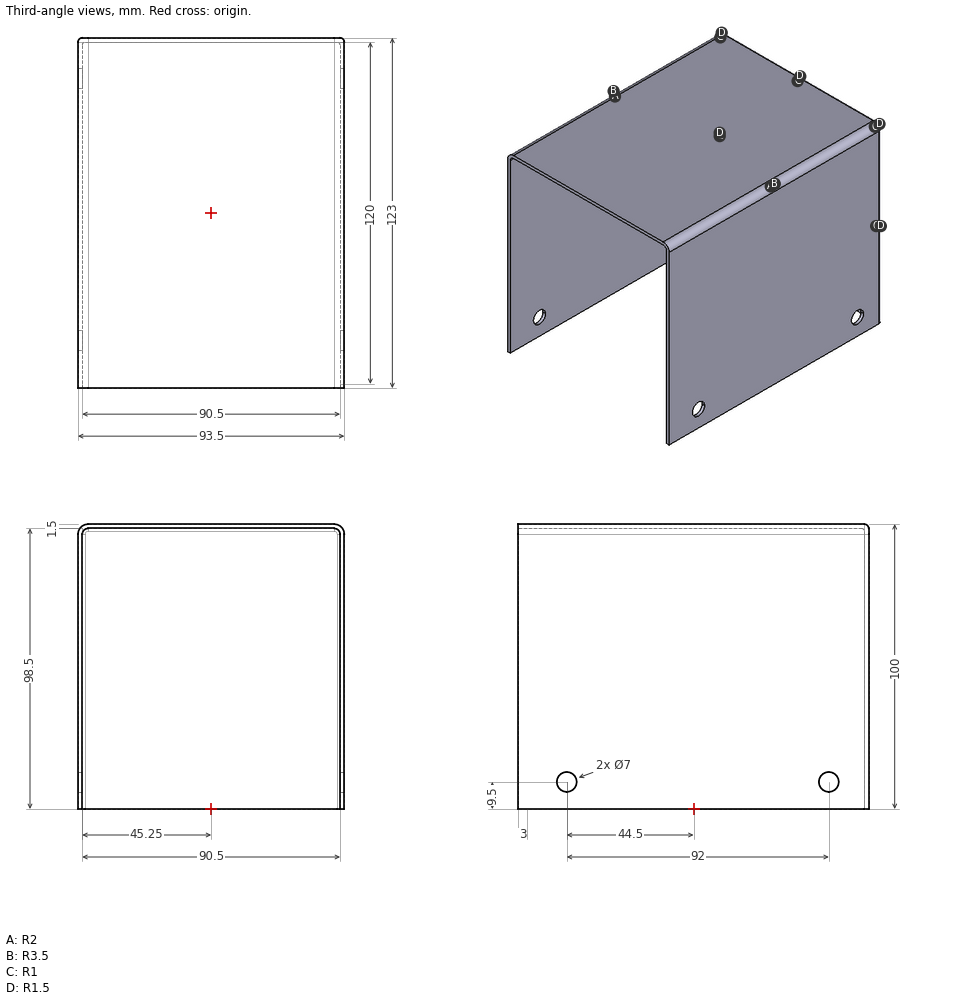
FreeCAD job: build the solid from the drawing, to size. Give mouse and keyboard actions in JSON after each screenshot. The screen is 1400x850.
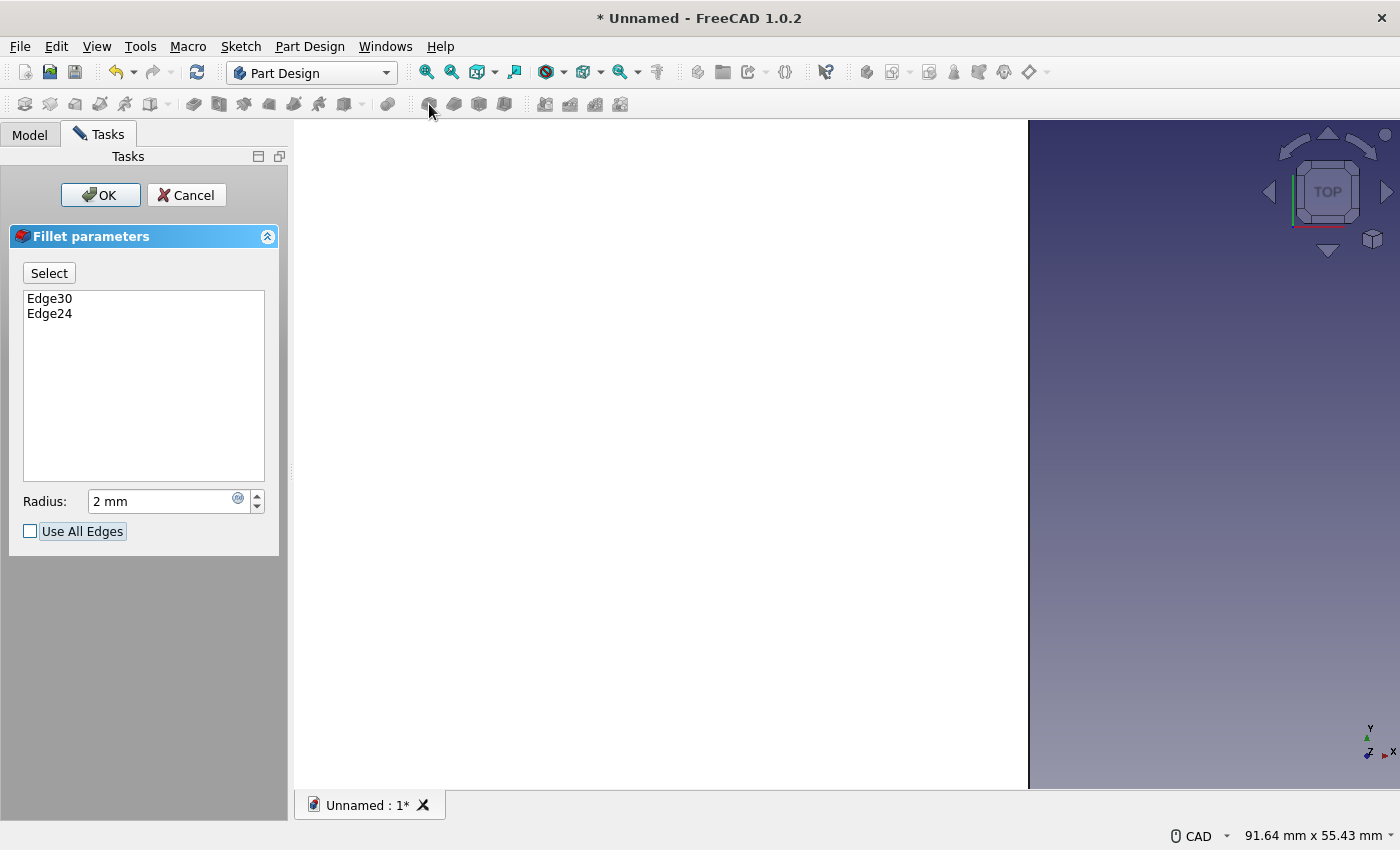
{"action": "left_click", "coordinate": [101, 195]}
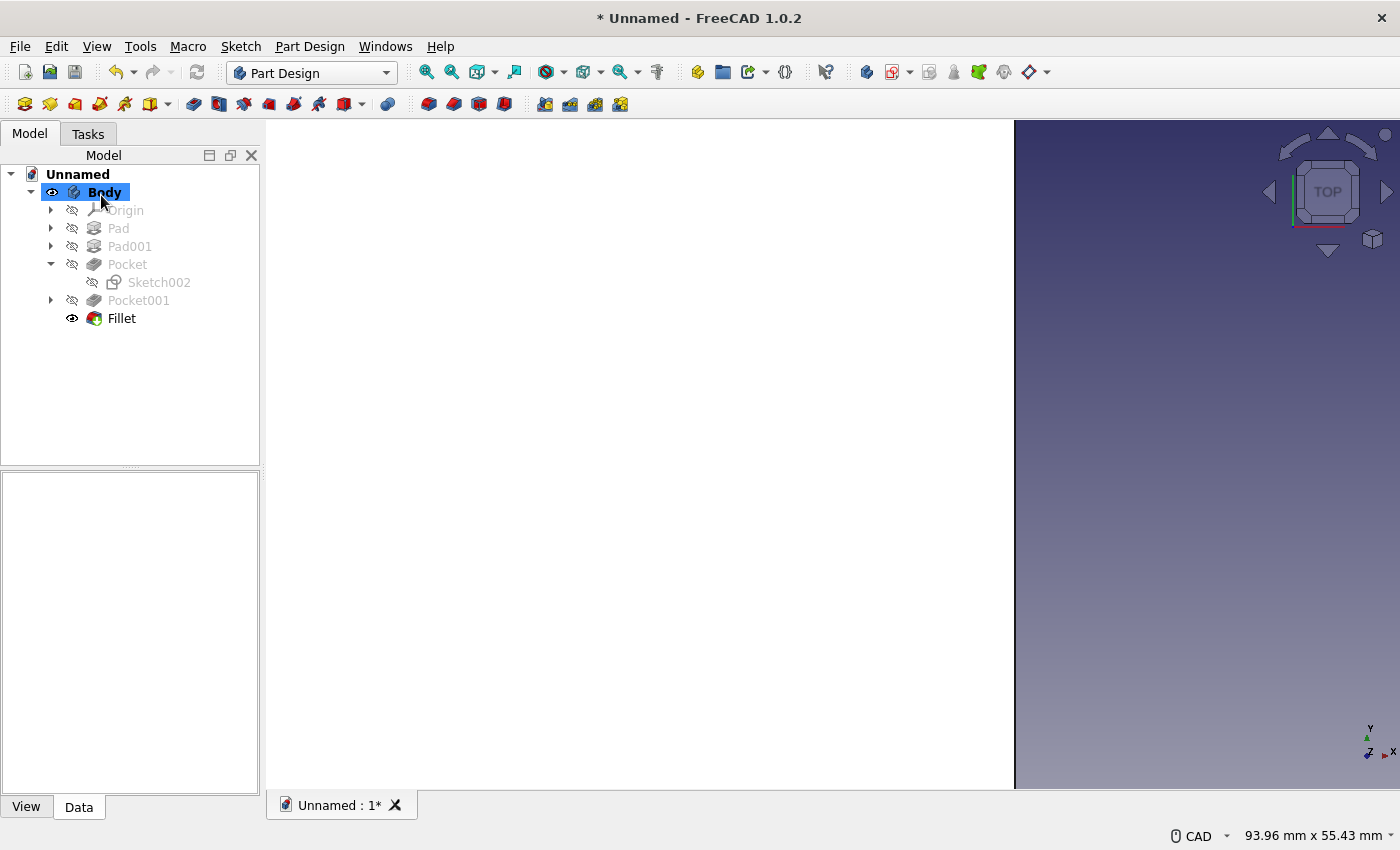
{"action": "left_click", "coordinate": [427, 72]}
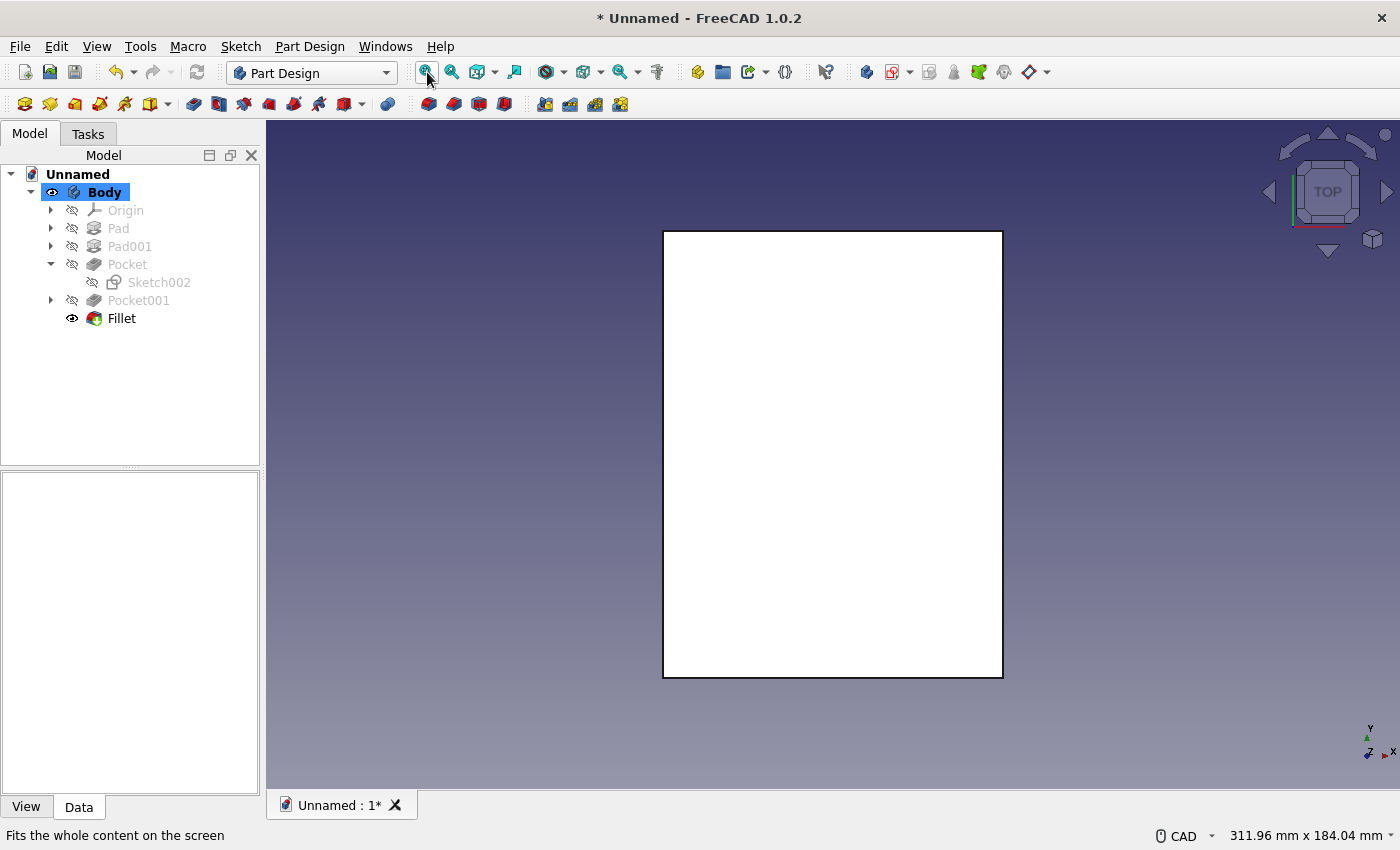
{"action": "left_click", "coordinate": [663, 453]}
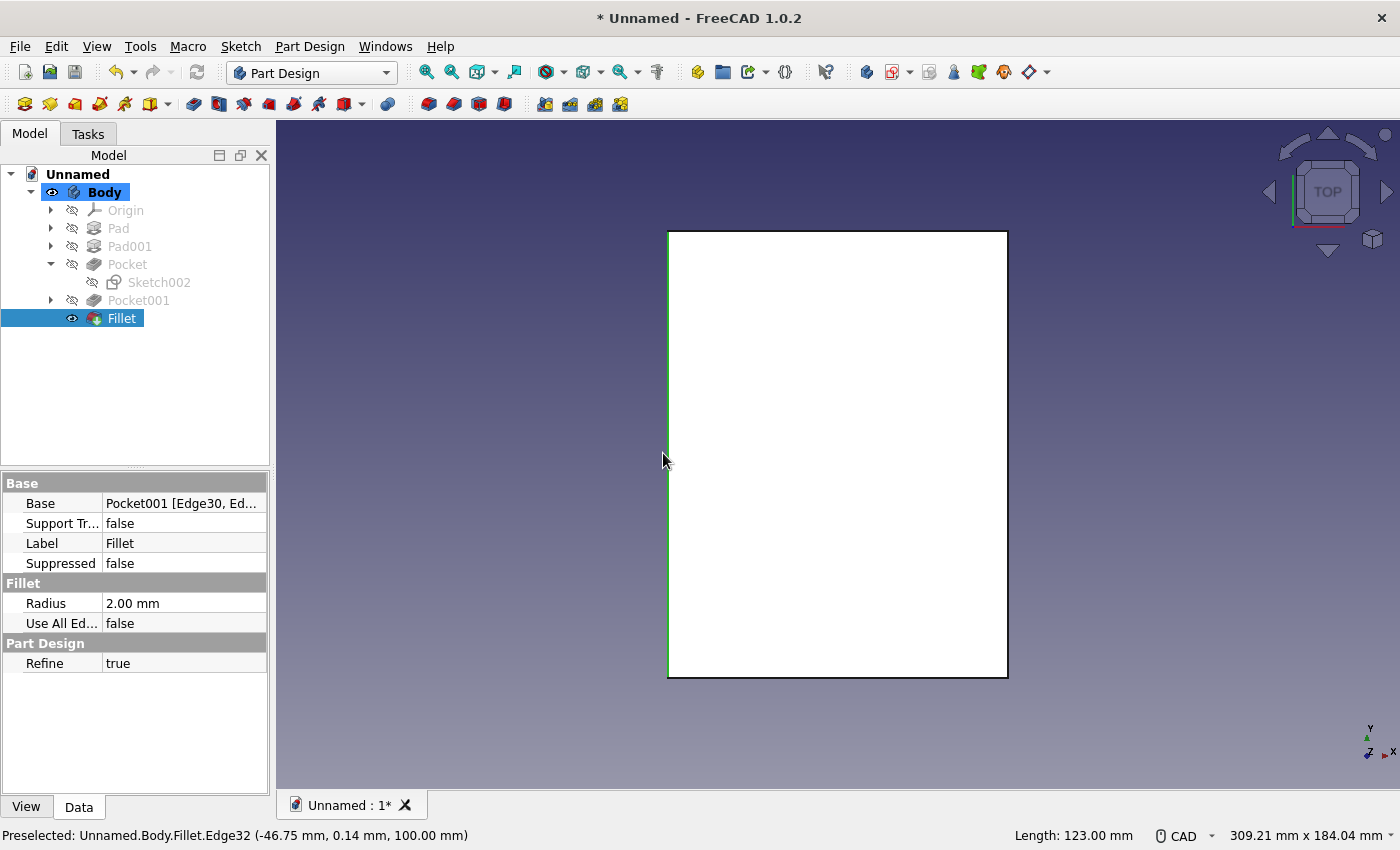
{"action": "left_click", "coordinate": [1008, 453], "text": "ctrl"}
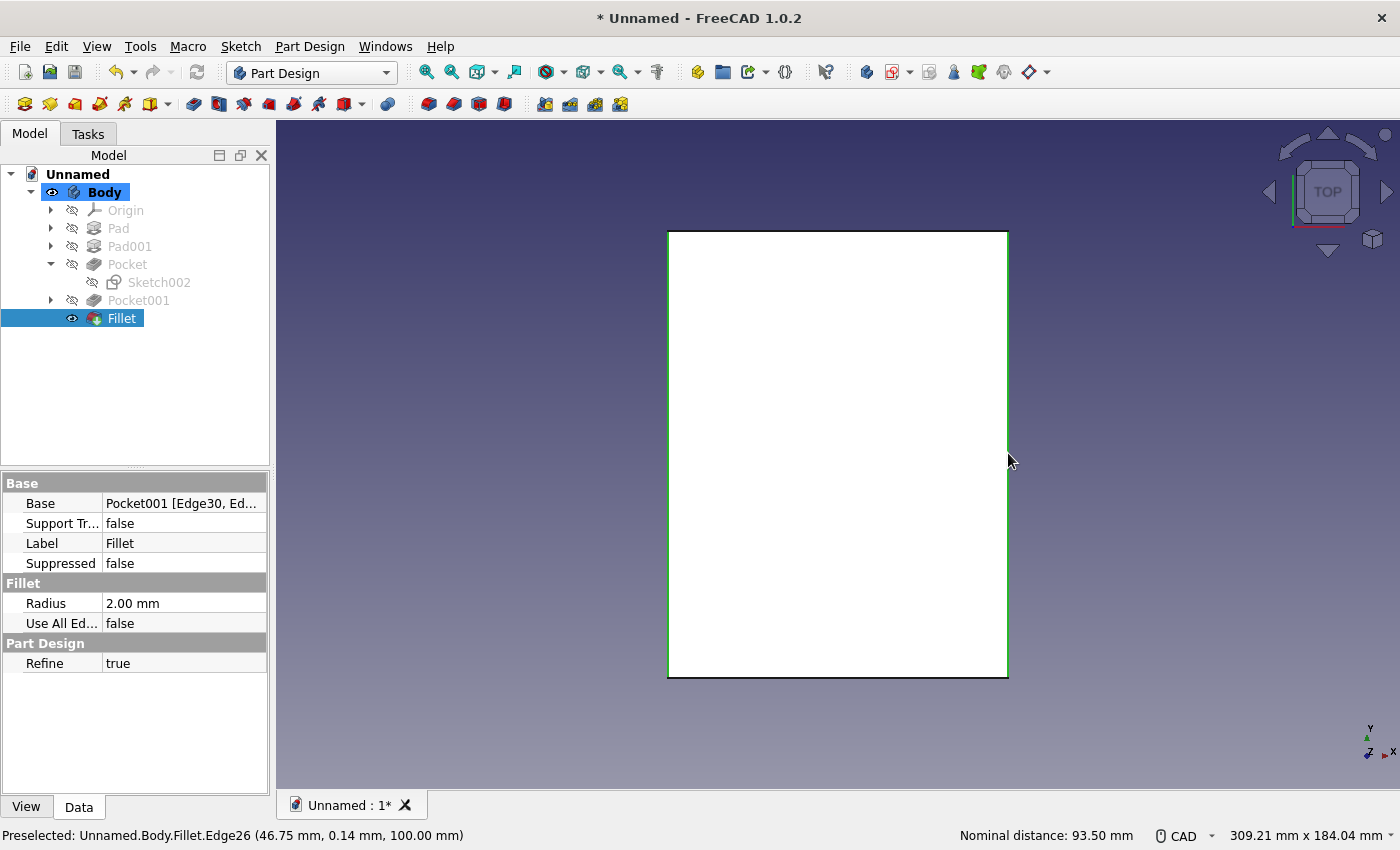
{"action": "left_click", "coordinate": [429, 104]}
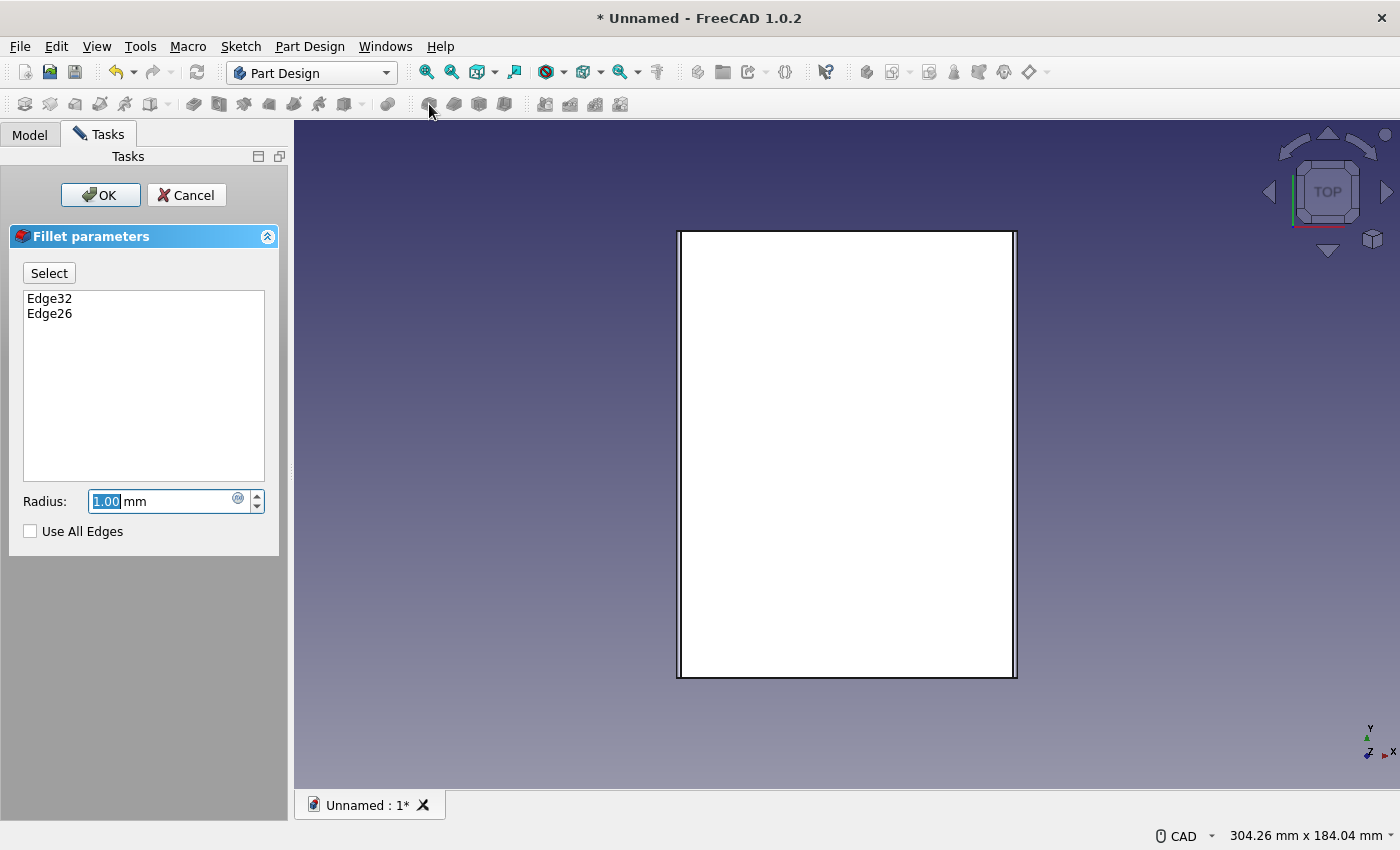
{"action": "type", "text": "3.5"}
{"action": "key", "text": "Tab"}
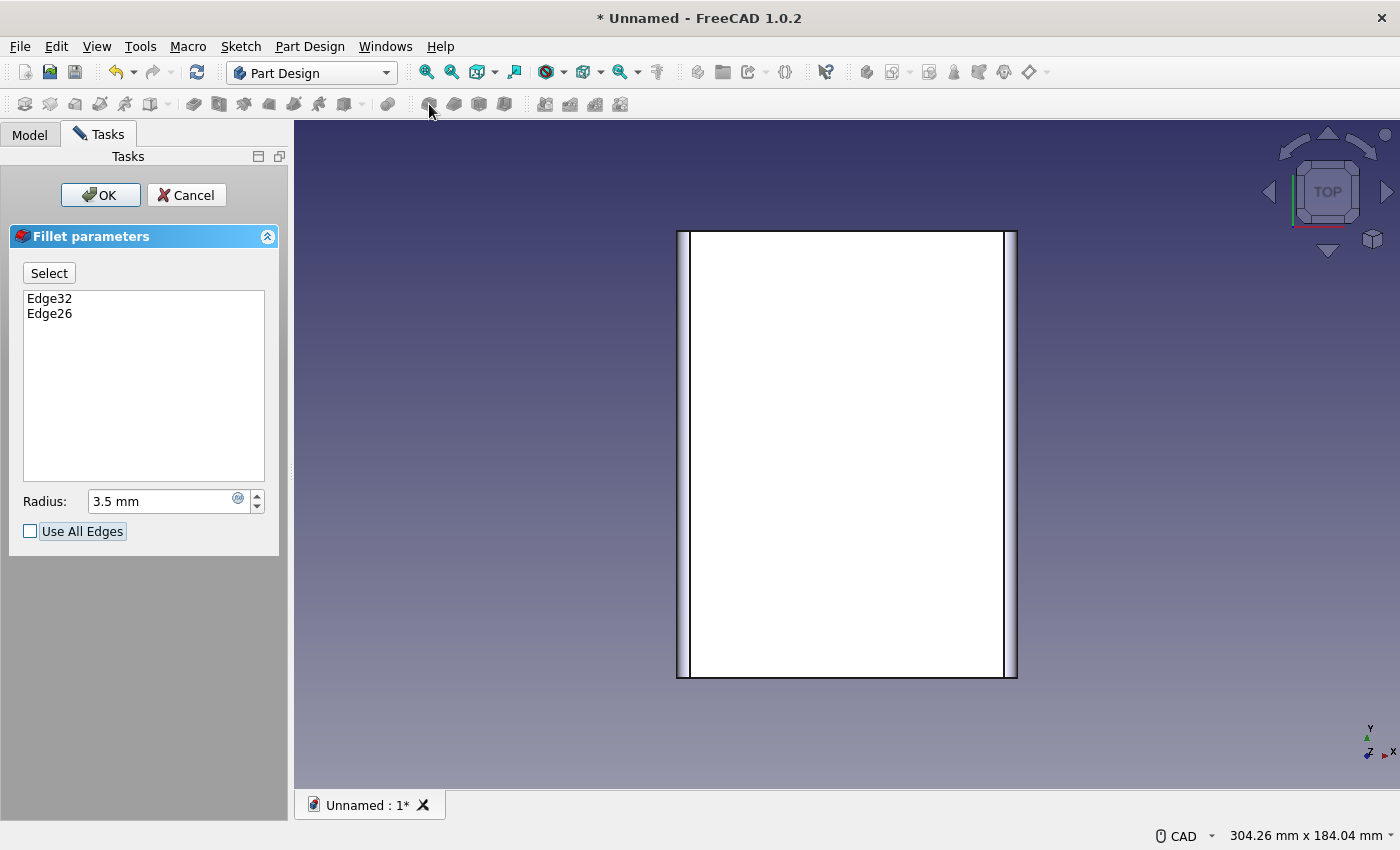
{"action": "left_click", "coordinate": [101, 195]}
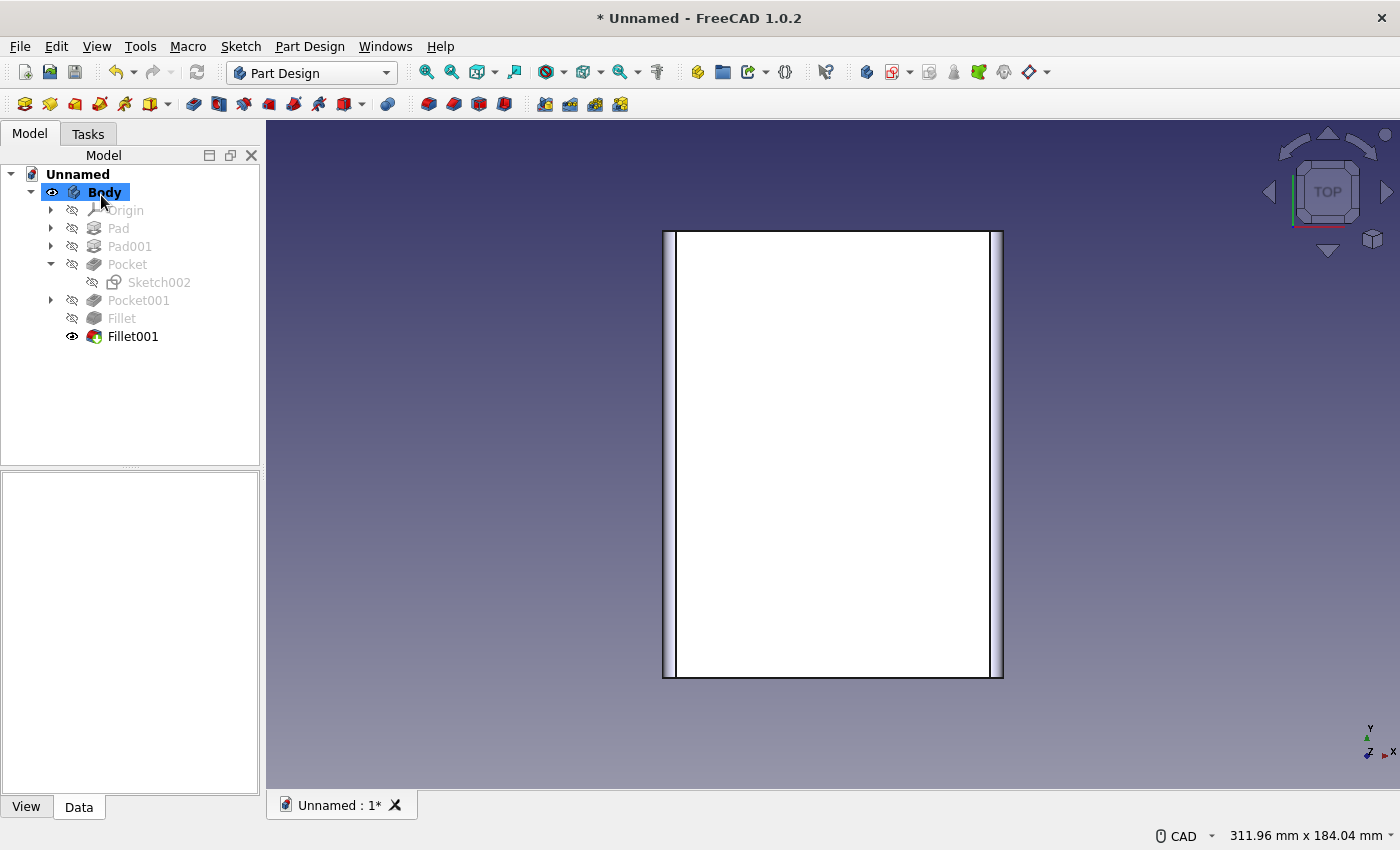
{"action": "key", "text": "0"}